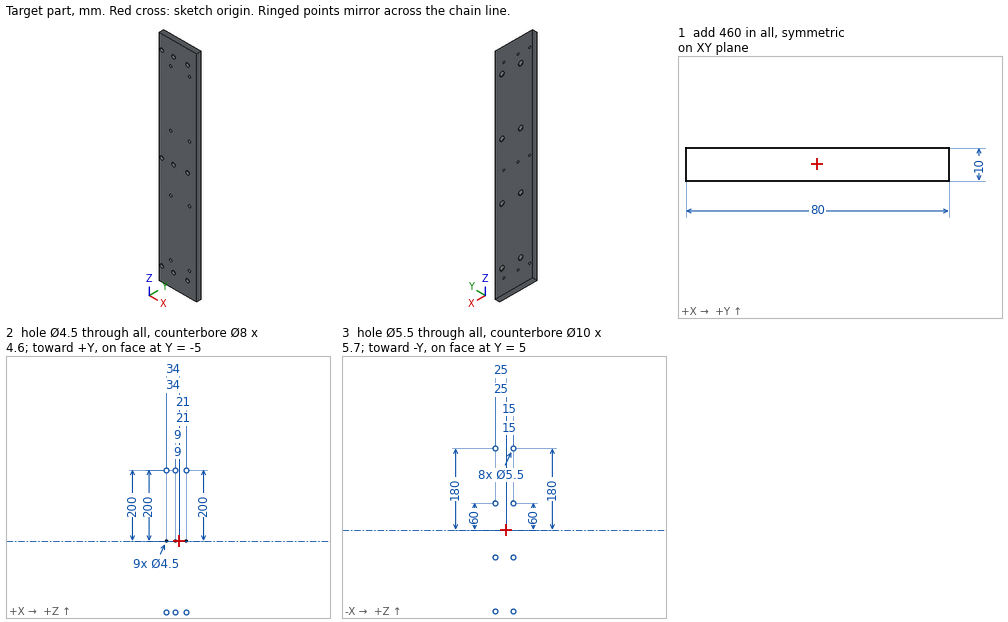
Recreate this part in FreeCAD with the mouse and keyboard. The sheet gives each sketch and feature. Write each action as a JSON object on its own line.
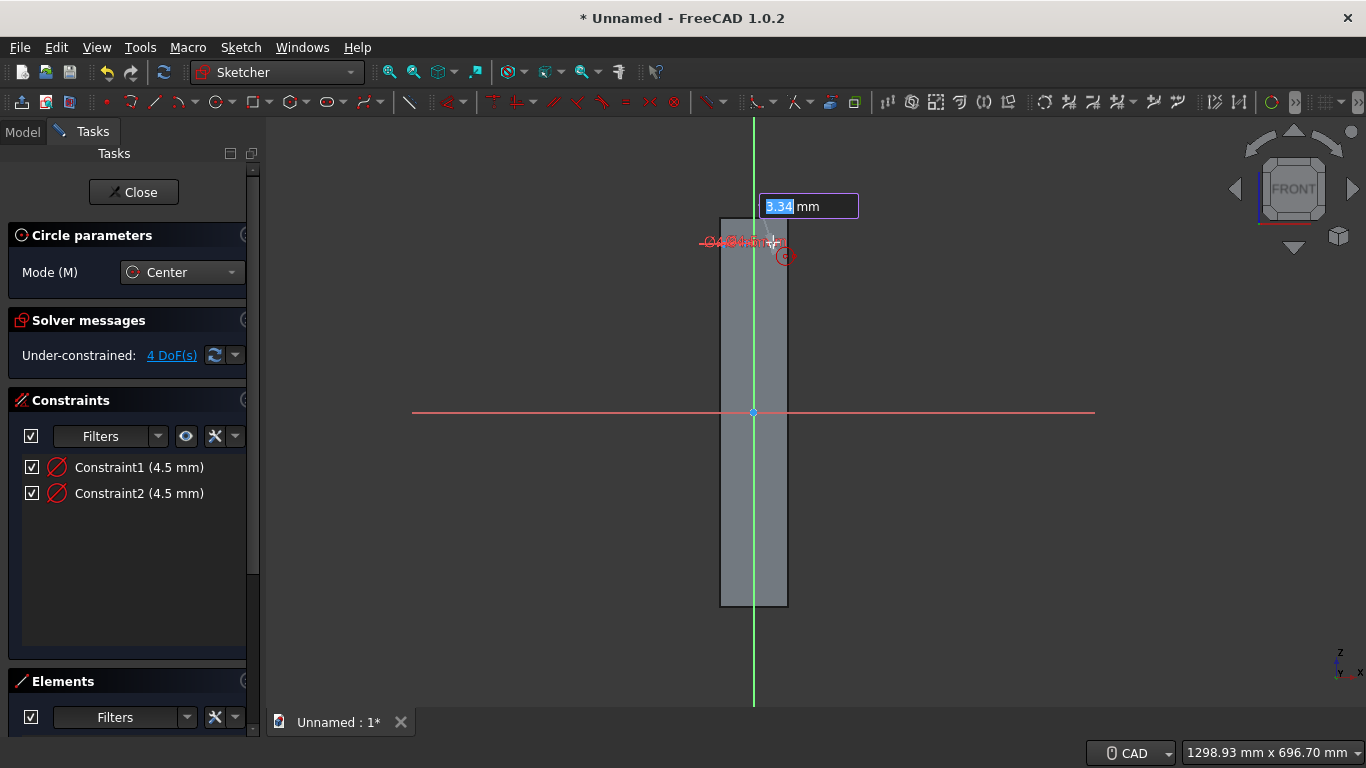
{"action": "type", "text": "4.5"}
{"action": "key", "text": "Return"}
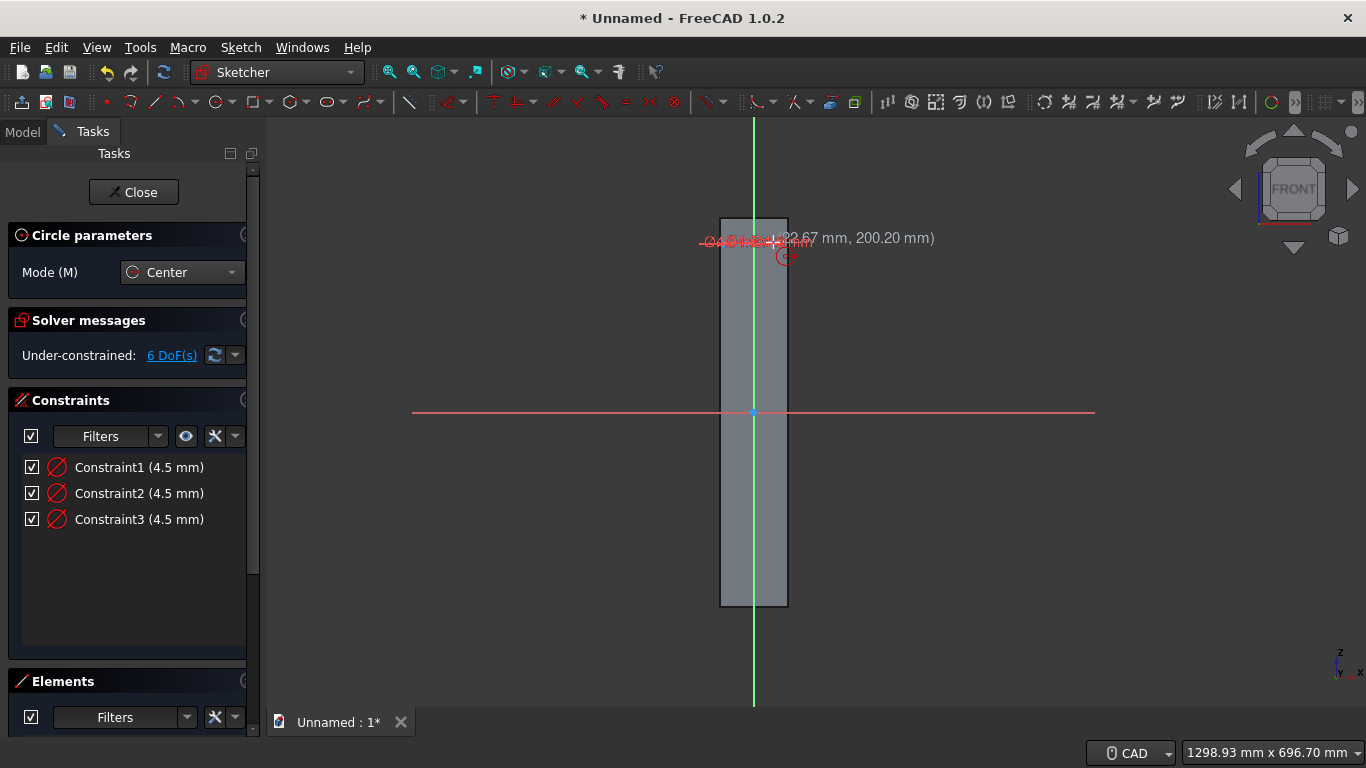
{"action": "scroll", "coordinate": [725, 413], "scroll_direction": "up", "scroll_amount": 13}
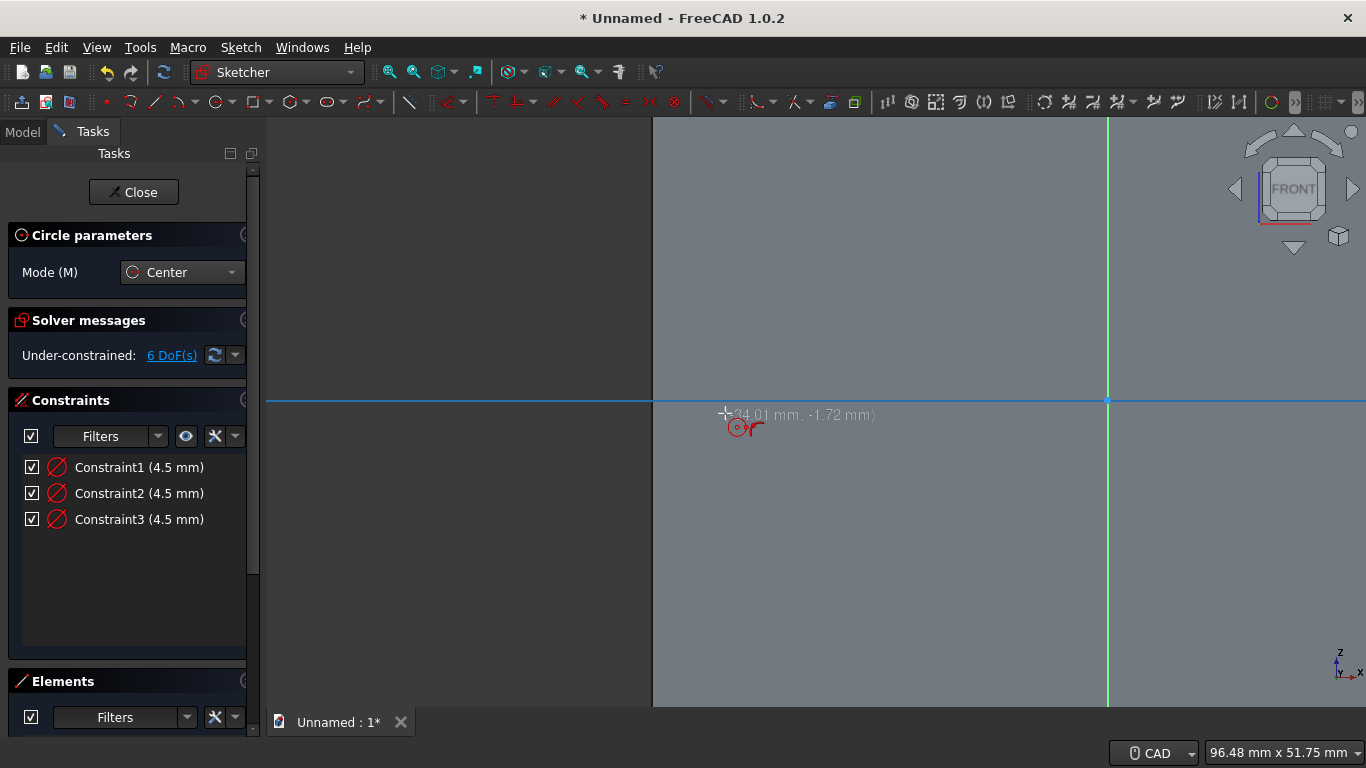
{"action": "scroll", "coordinate": [725, 413], "scroll_direction": "down", "scroll_amount": 13}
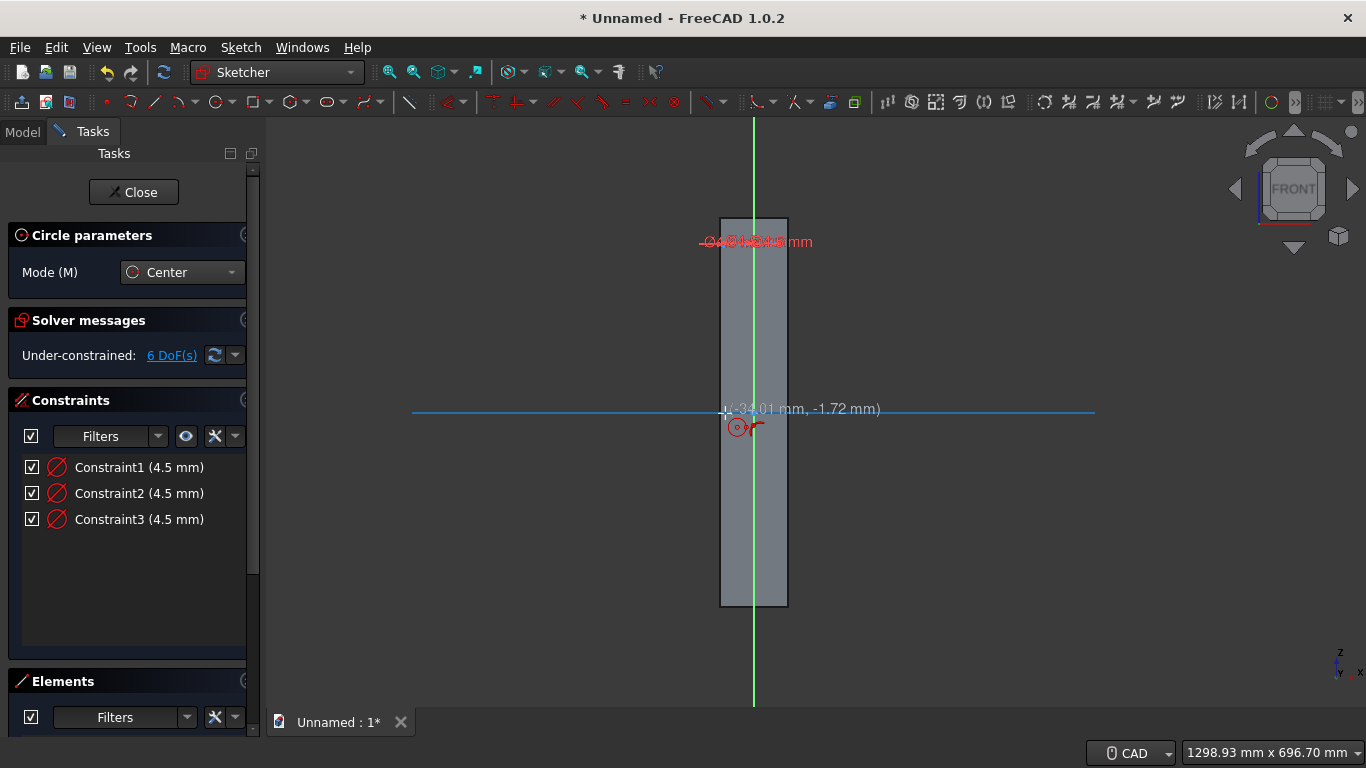
{"action": "left_click", "coordinate": [725, 413]}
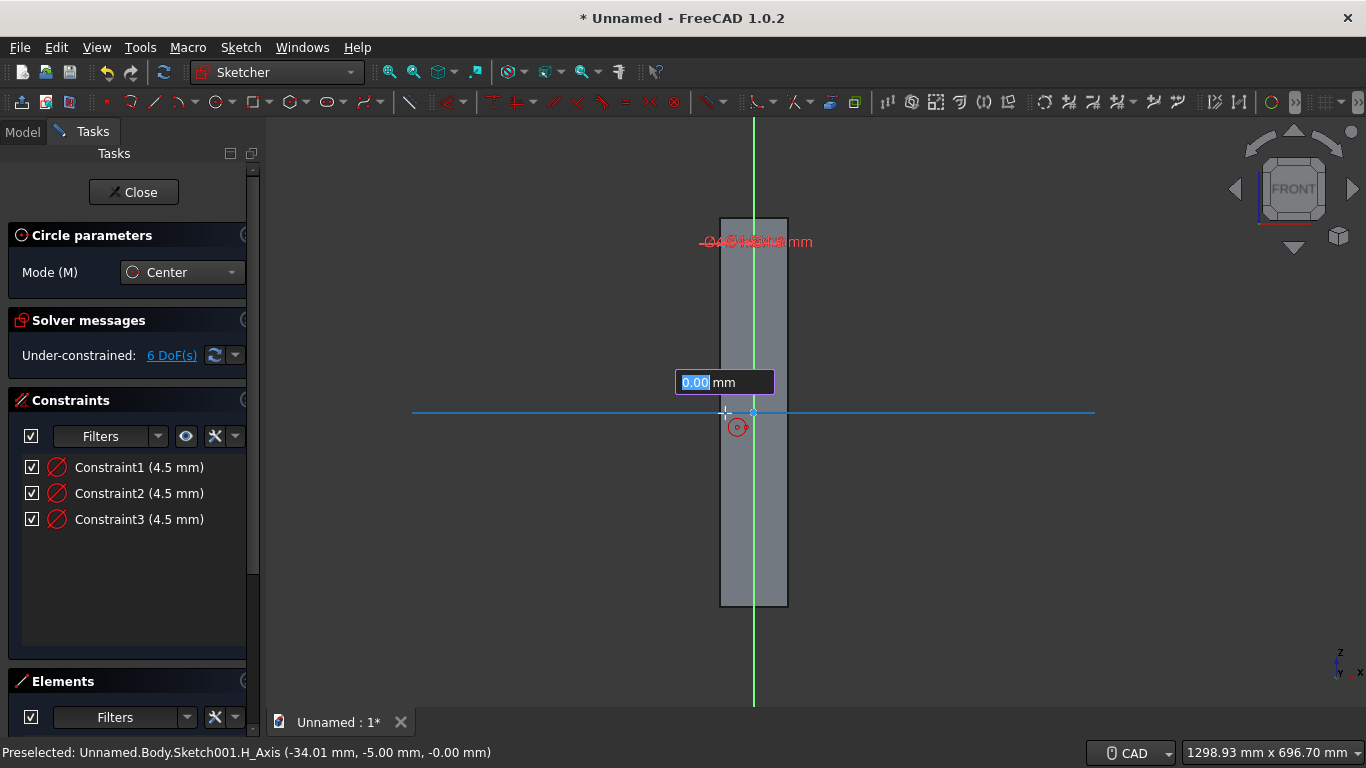
{"action": "scroll", "coordinate": [724, 414], "scroll_direction": "up", "scroll_amount": 11}
{"action": "mouse_move", "coordinate": [724, 413]}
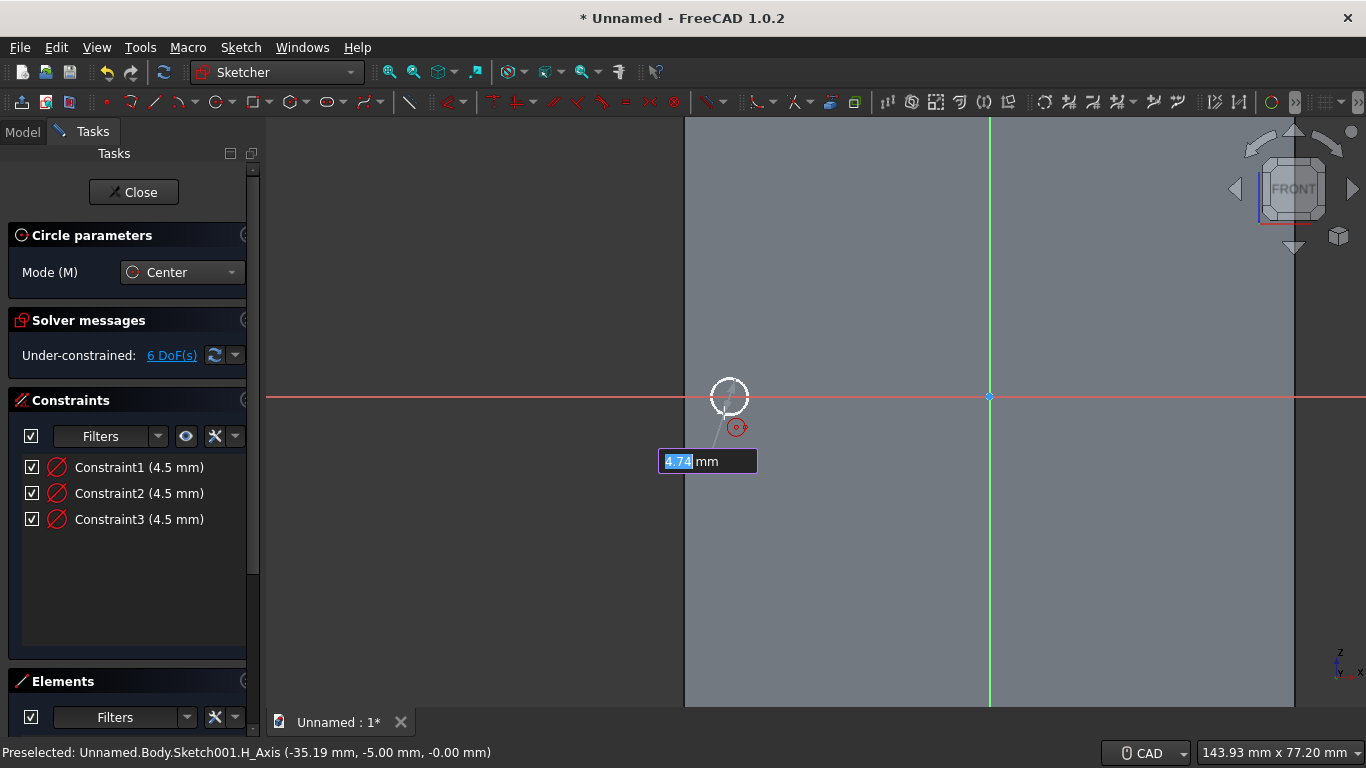
{"action": "type", "text": "4.5"}
{"action": "key", "text": "Return"}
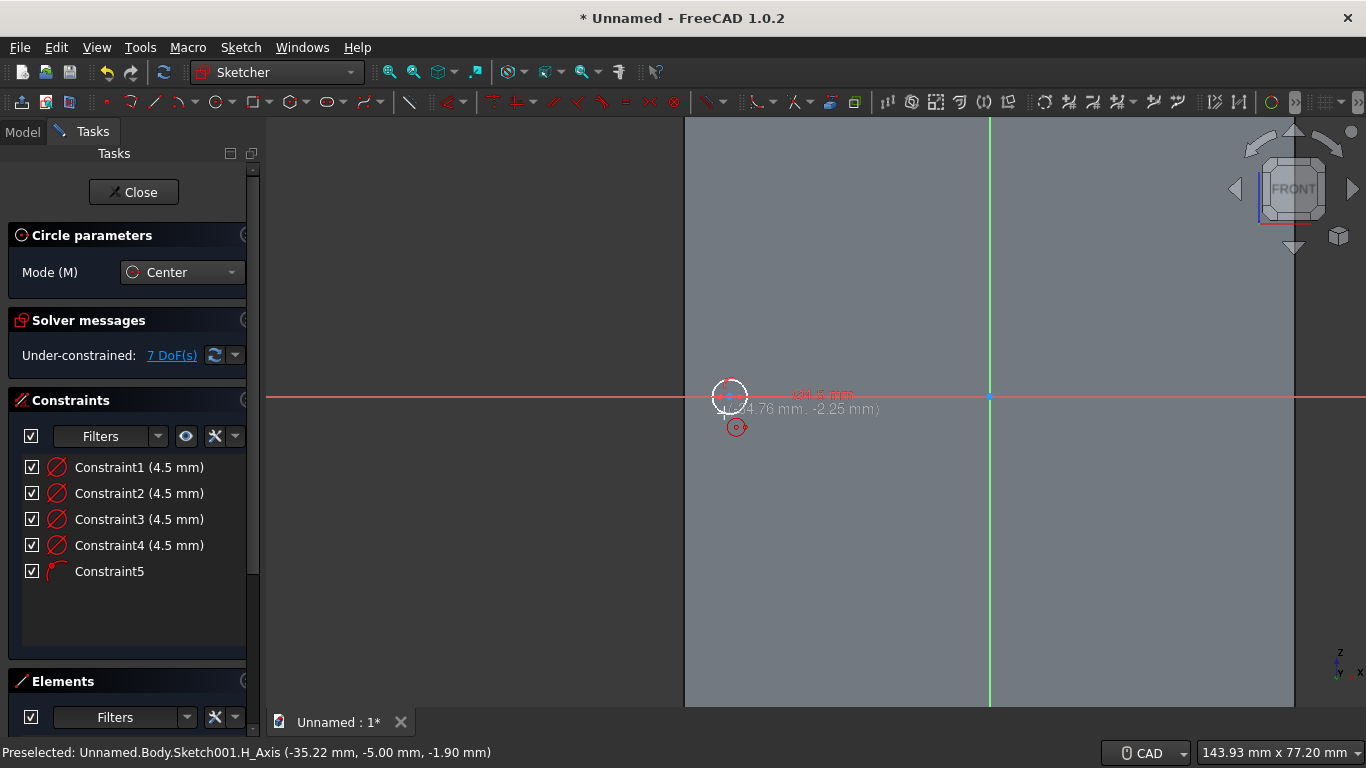
{"action": "scroll", "coordinate": [921, 397], "scroll_direction": "up", "scroll_amount": 2}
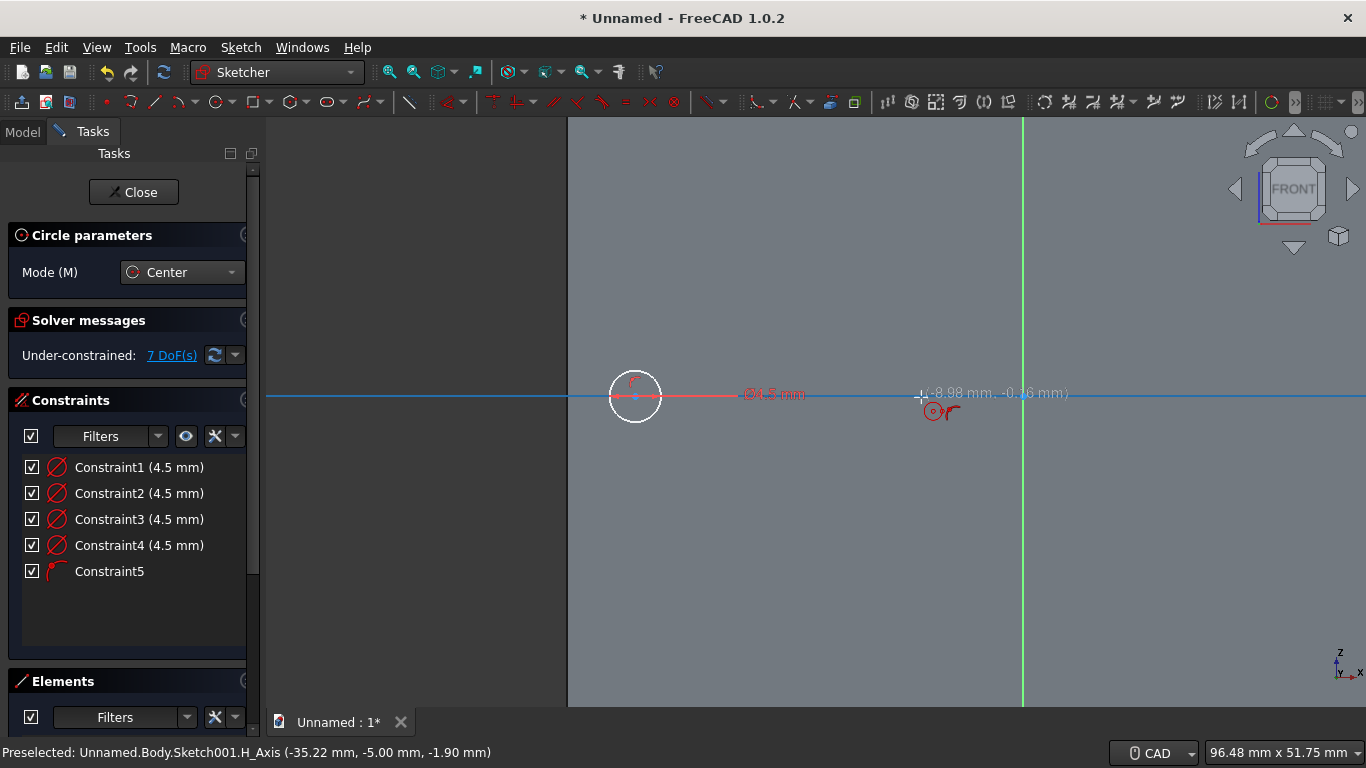
{"action": "scroll", "coordinate": [731, 413], "scroll_direction": "down", "scroll_amount": 13}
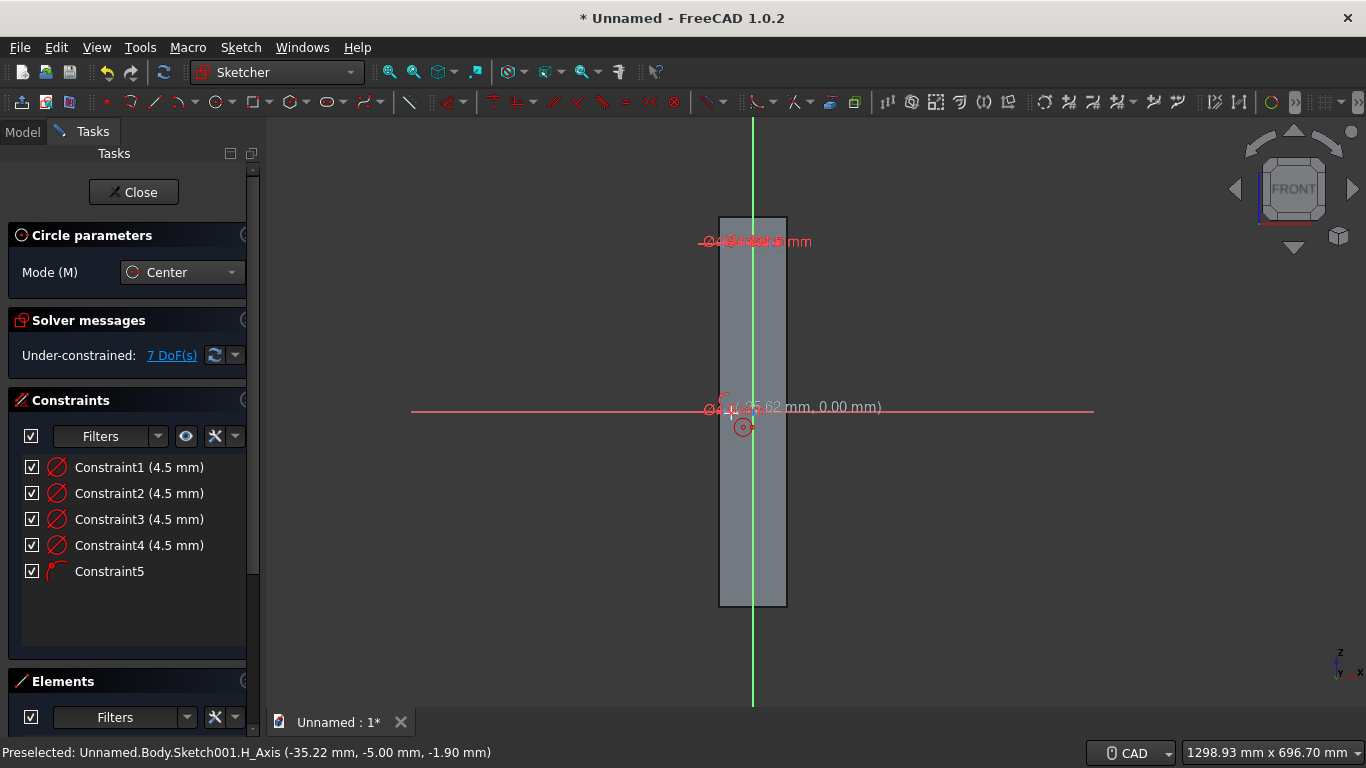
{"action": "scroll", "coordinate": [745, 412], "scroll_direction": "up", "scroll_amount": 4}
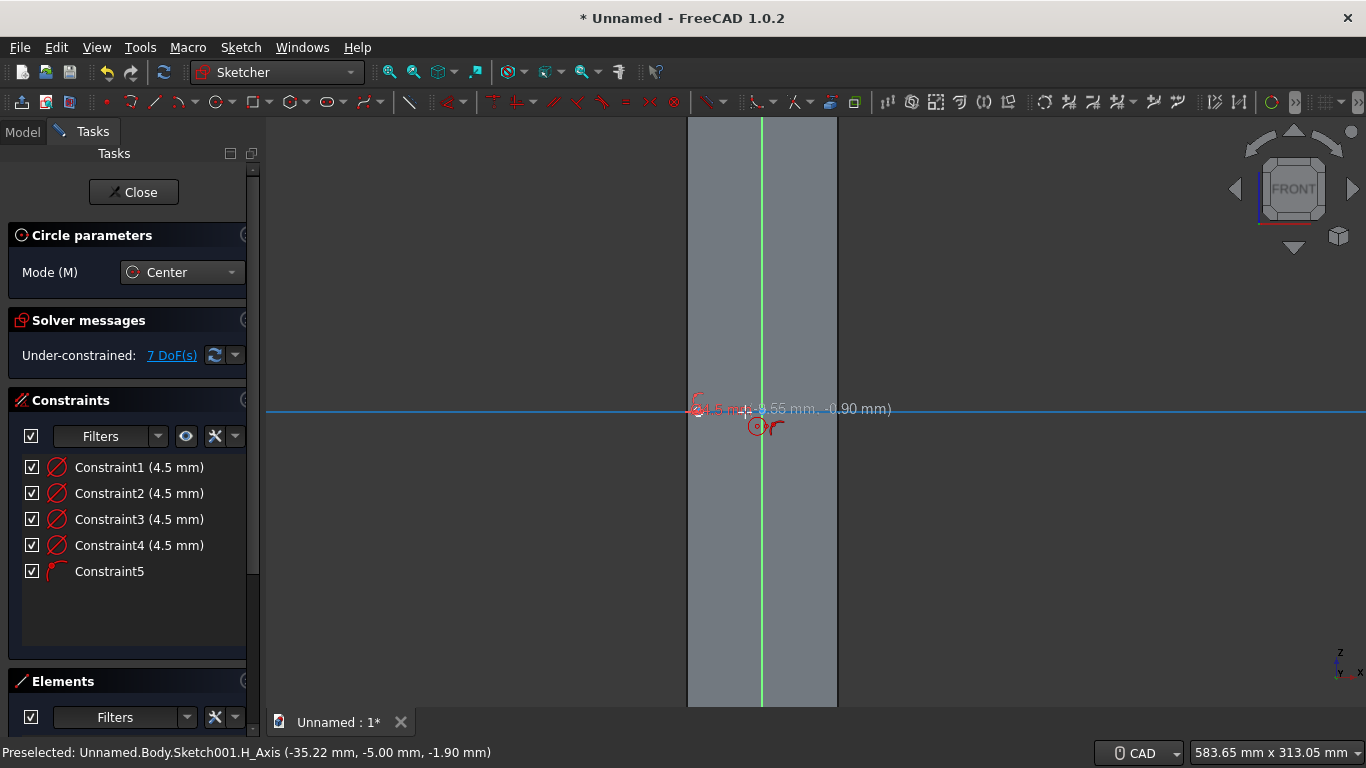
{"action": "left_click", "coordinate": [745, 412]}